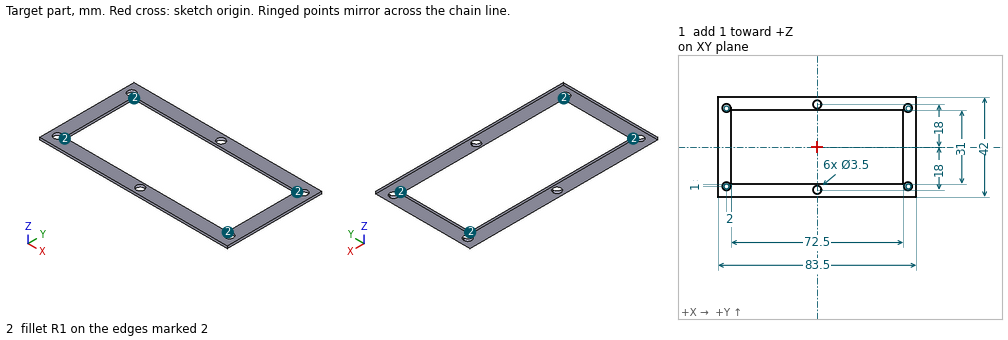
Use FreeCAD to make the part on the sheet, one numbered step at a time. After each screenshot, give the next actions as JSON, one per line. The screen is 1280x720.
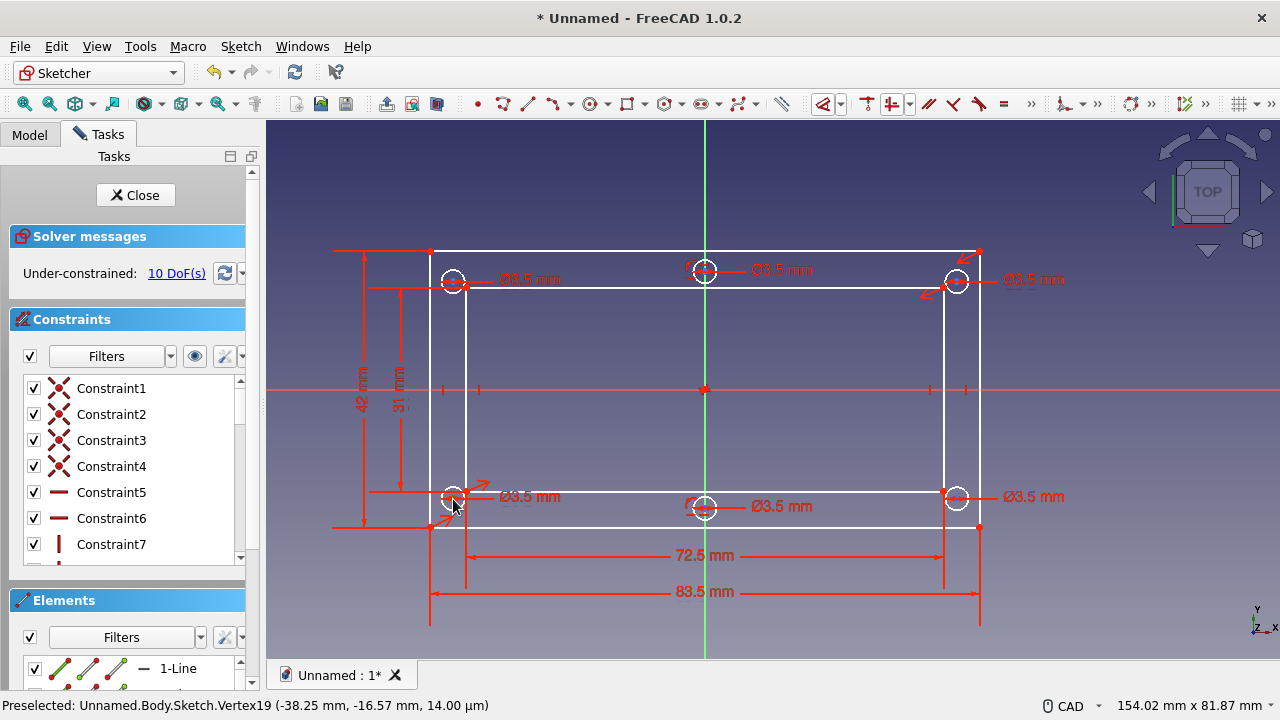
{"action": "left_click", "coordinate": [957, 499]}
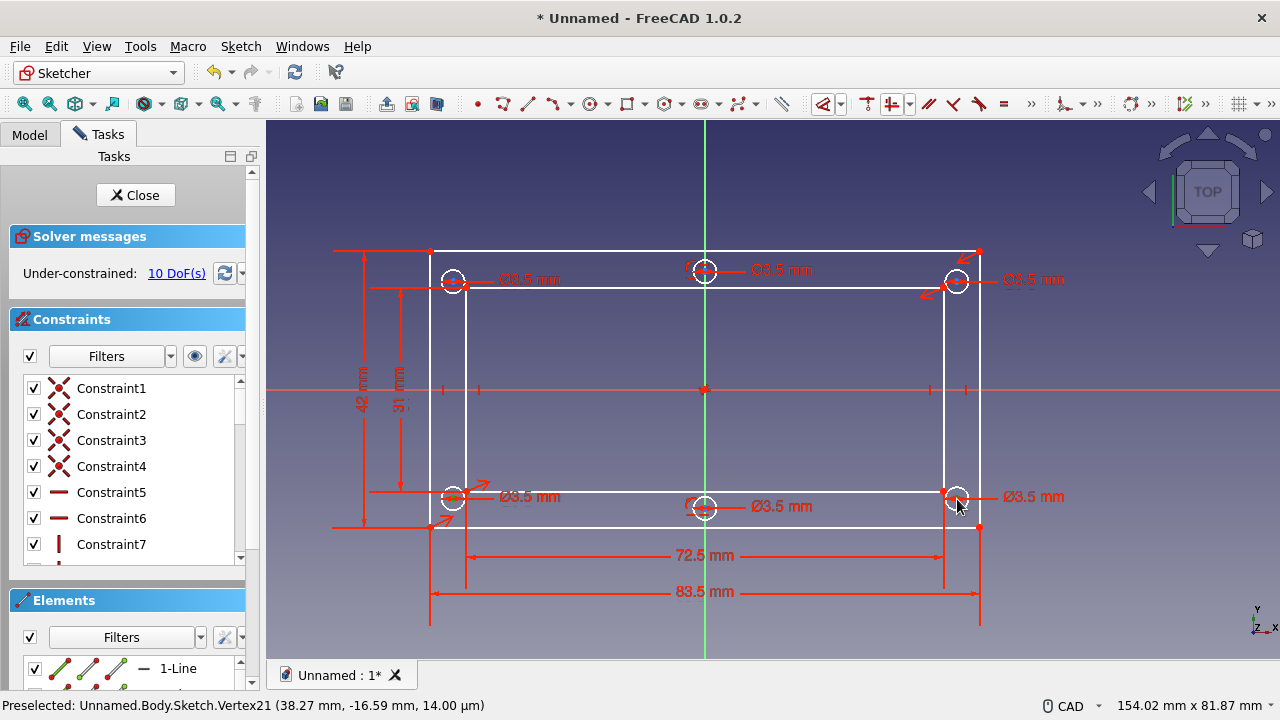
{"action": "left_click", "coordinate": [705, 458]}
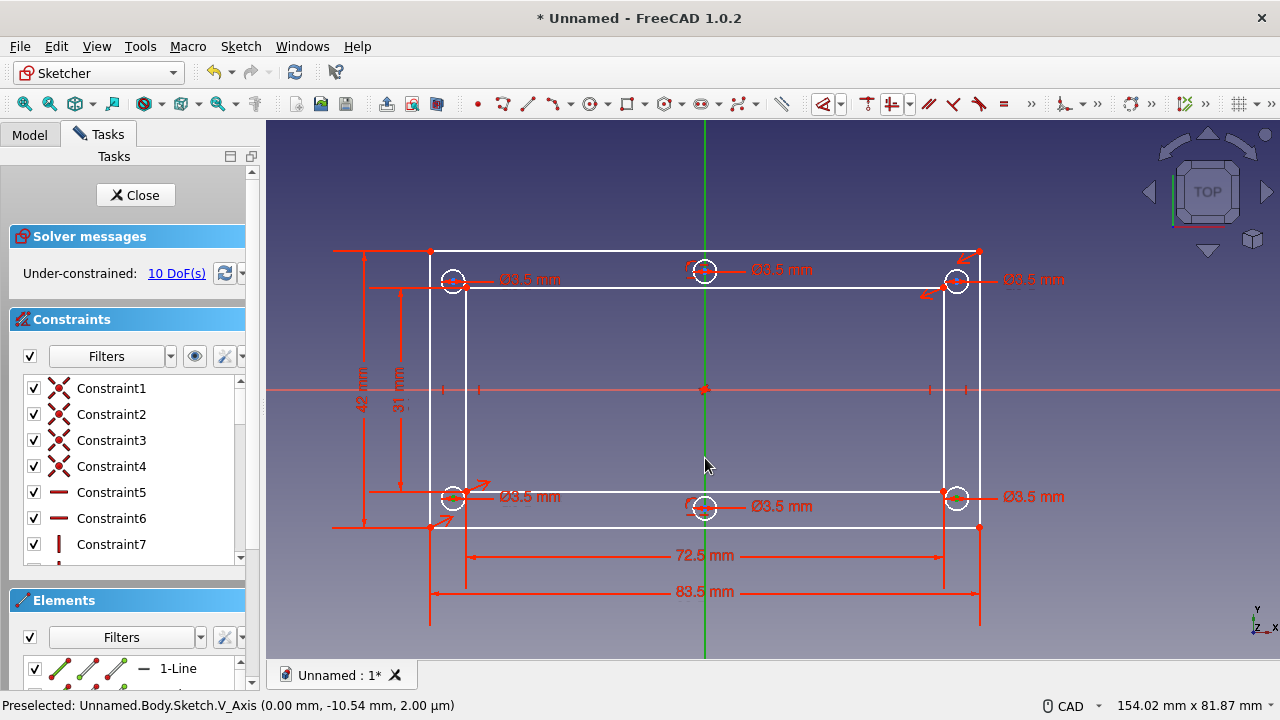
{"action": "key", "text": "s"}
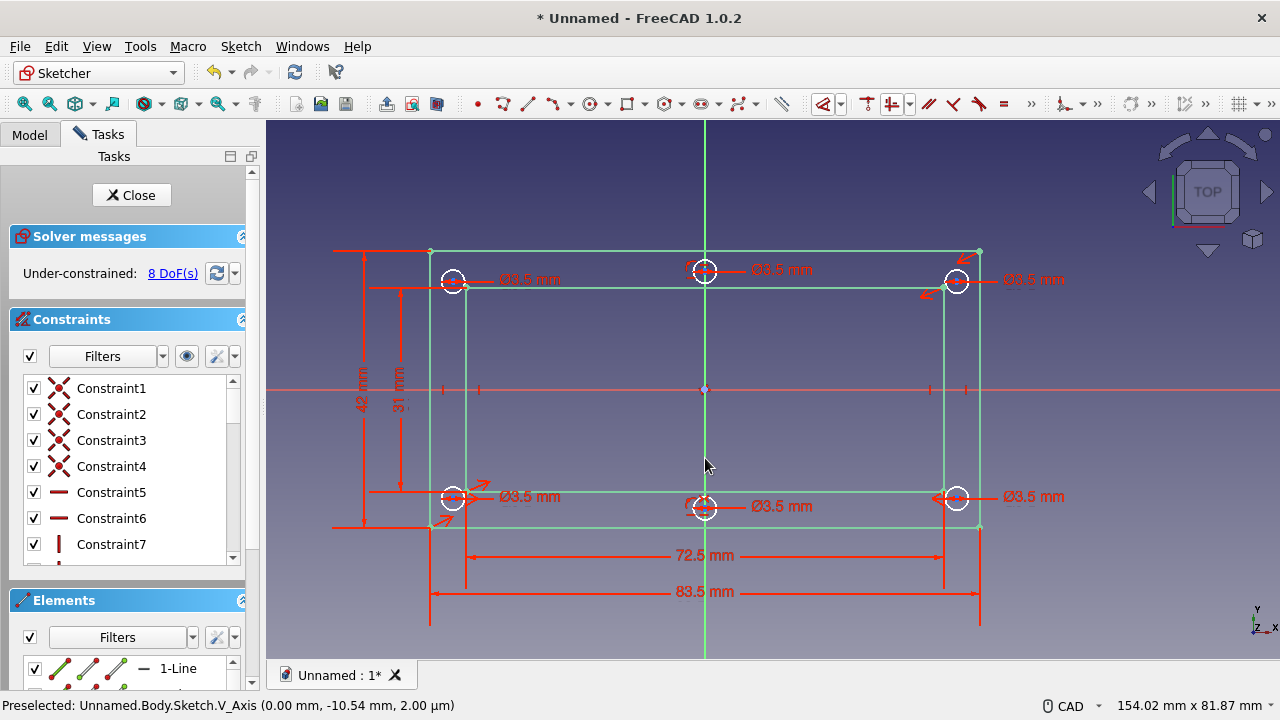
{"action": "left_click", "coordinate": [453, 499]}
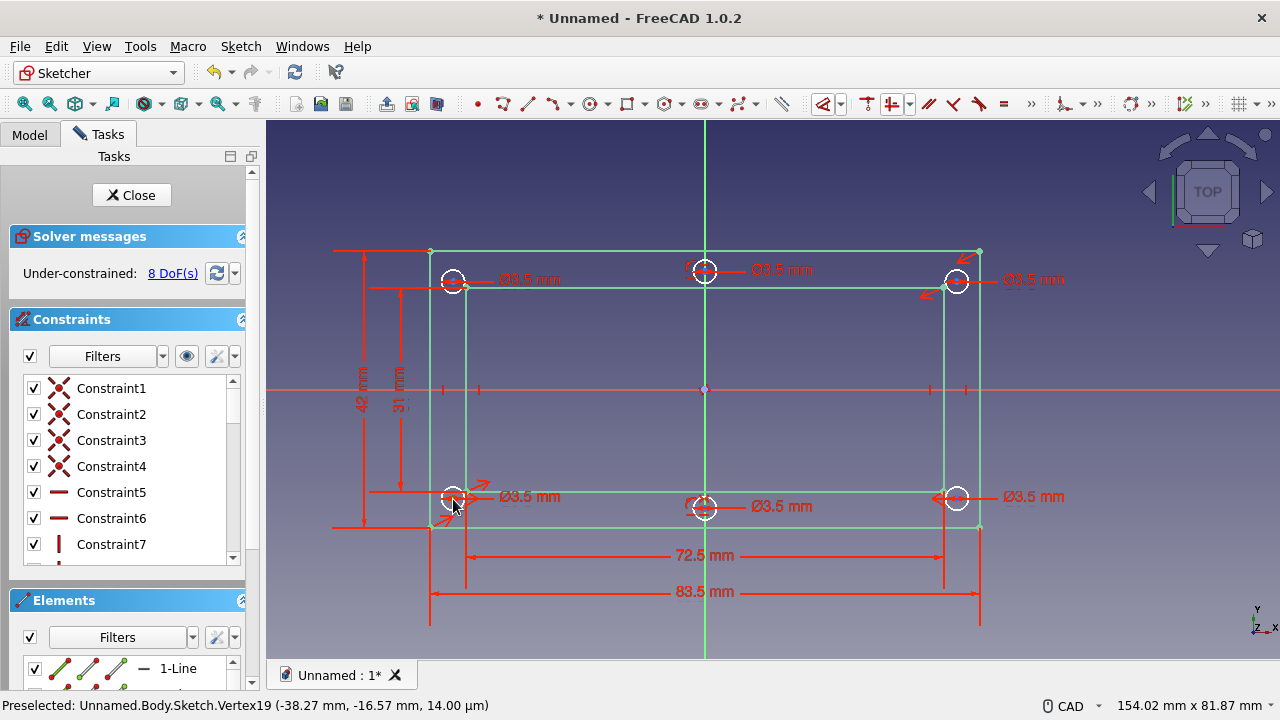
{"action": "left_click", "coordinate": [453, 282]}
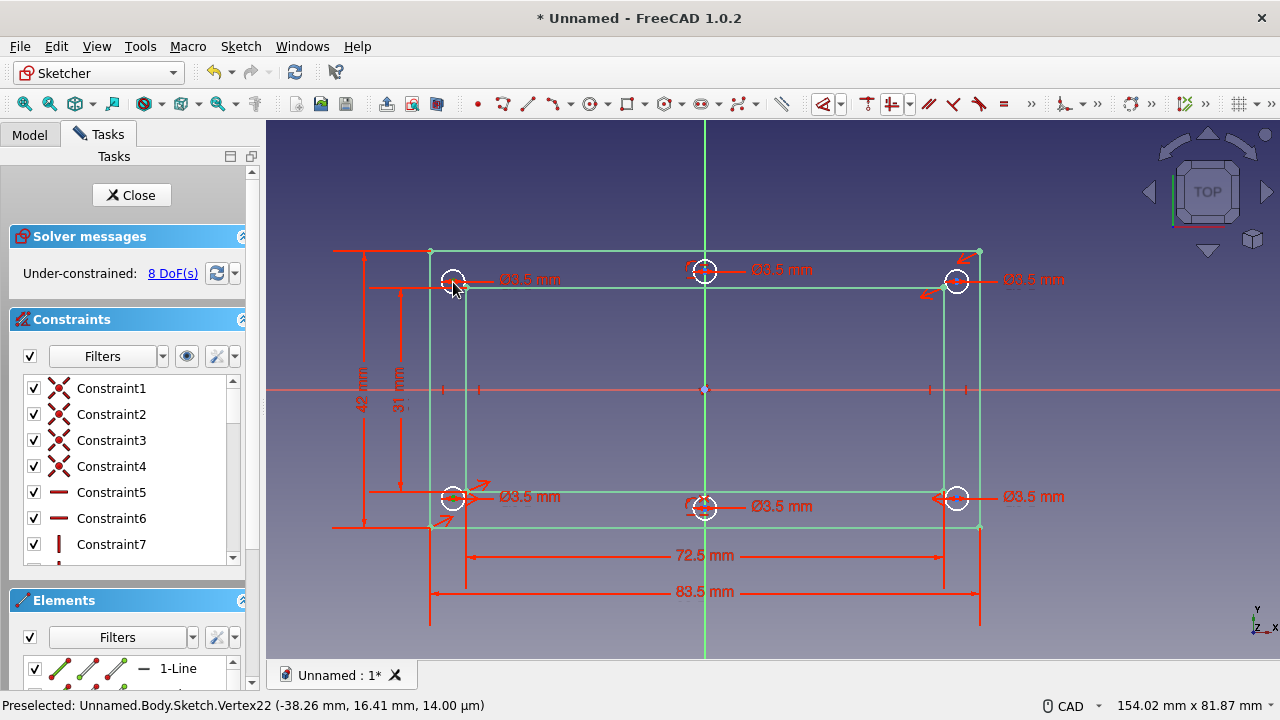
{"action": "left_click", "coordinate": [353, 390]}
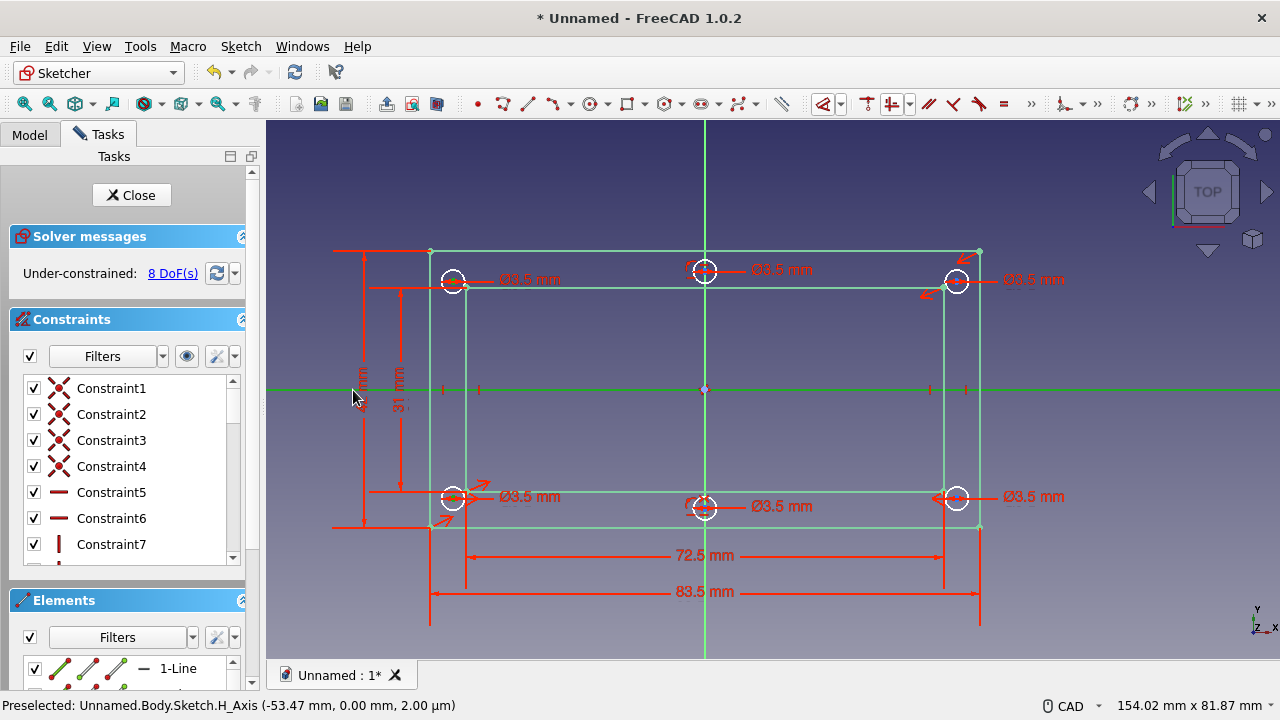
{"action": "key", "text": "s"}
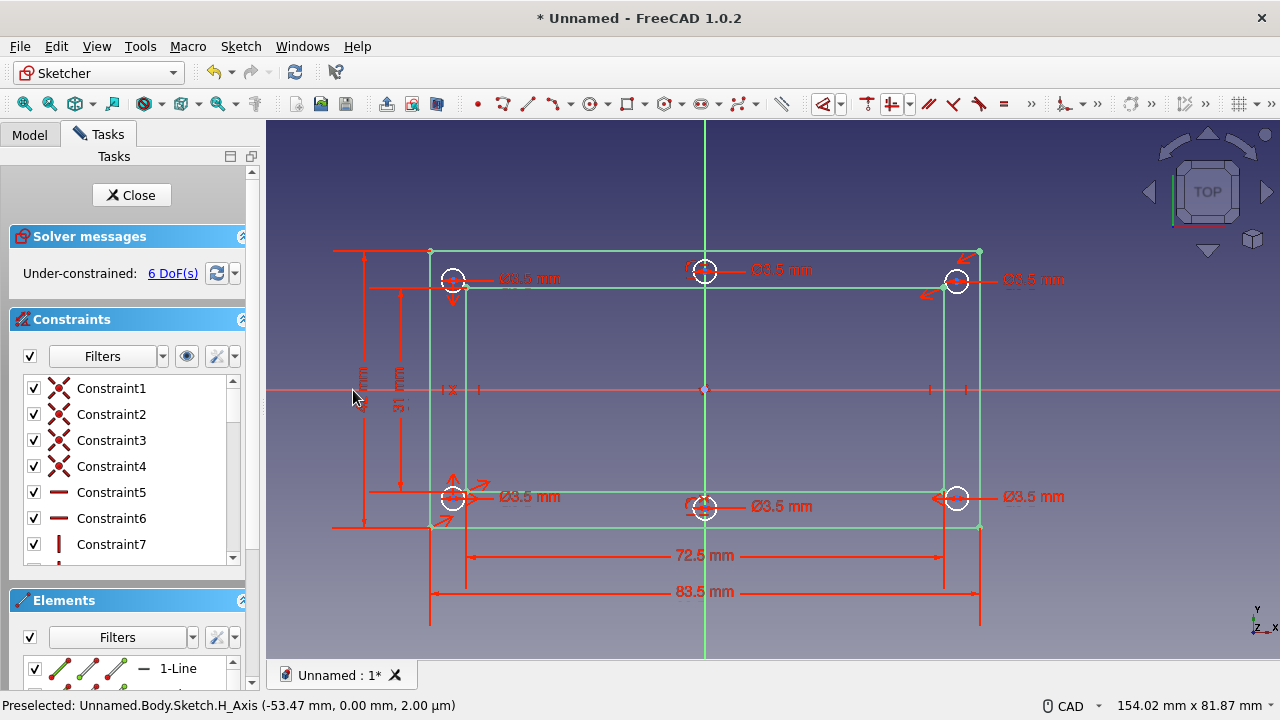
{"action": "left_click", "coordinate": [957, 499]}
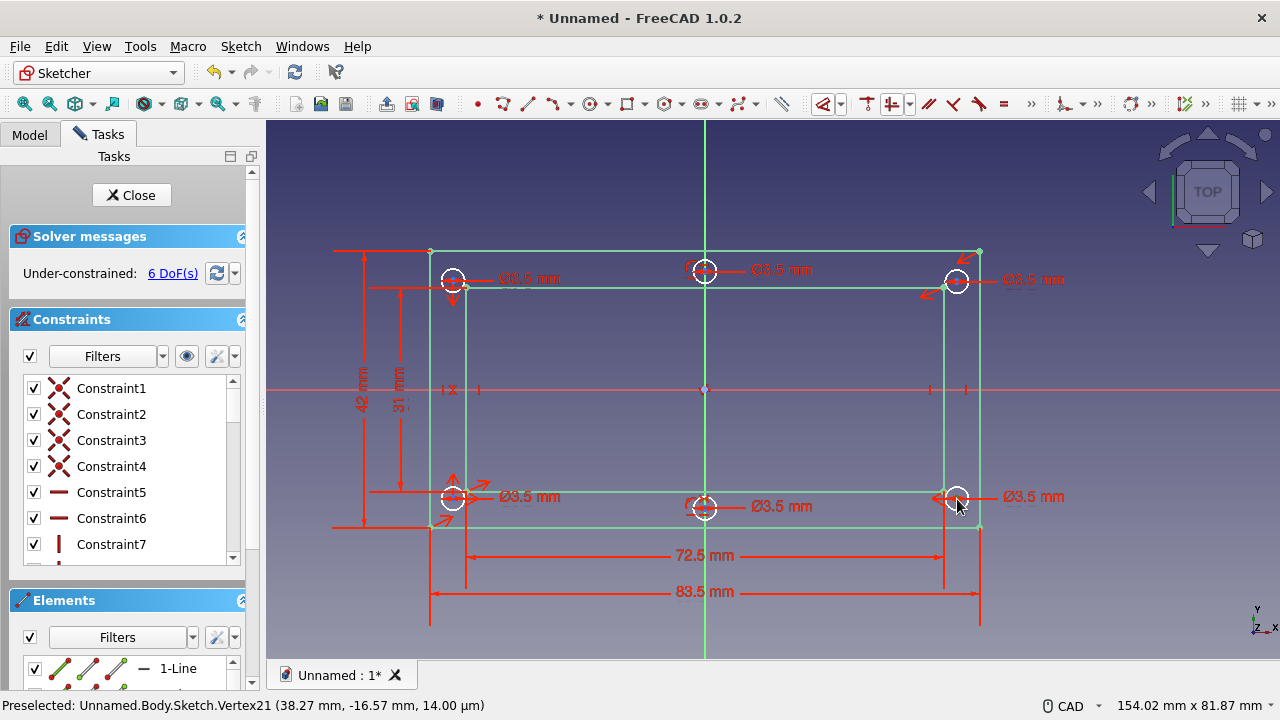
{"action": "left_click", "coordinate": [957, 282]}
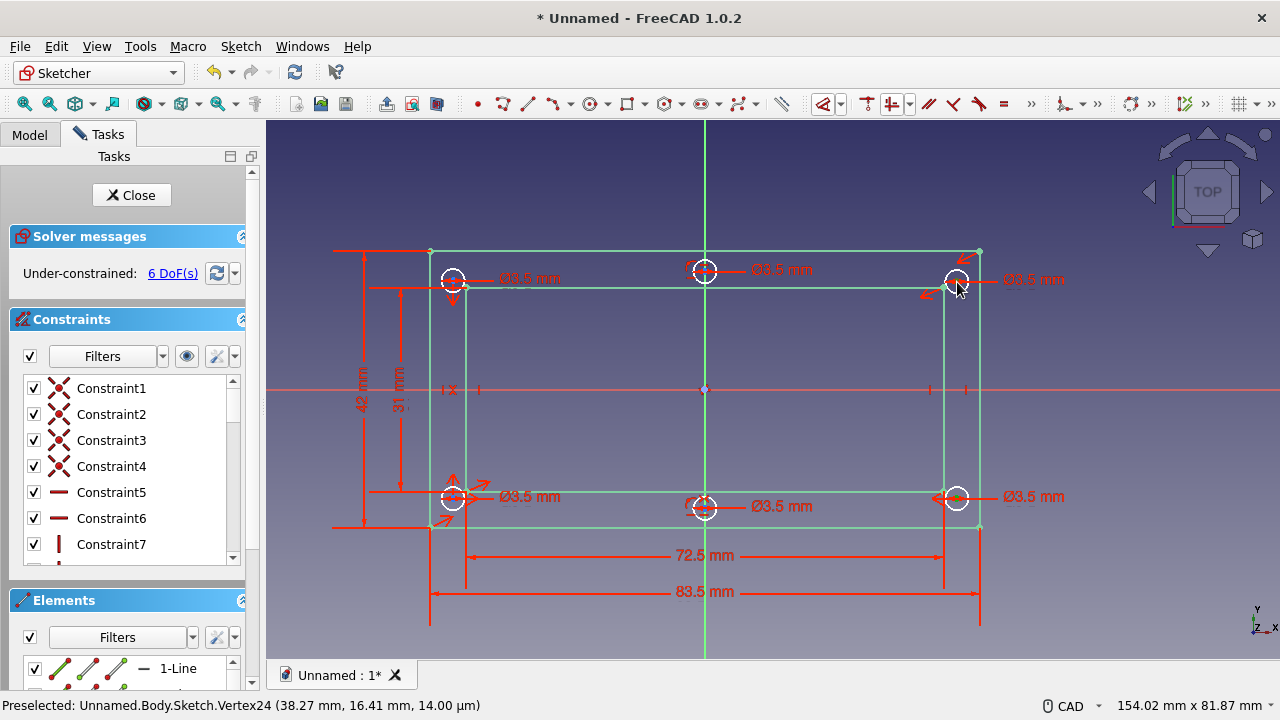
{"action": "left_click", "coordinate": [353, 390]}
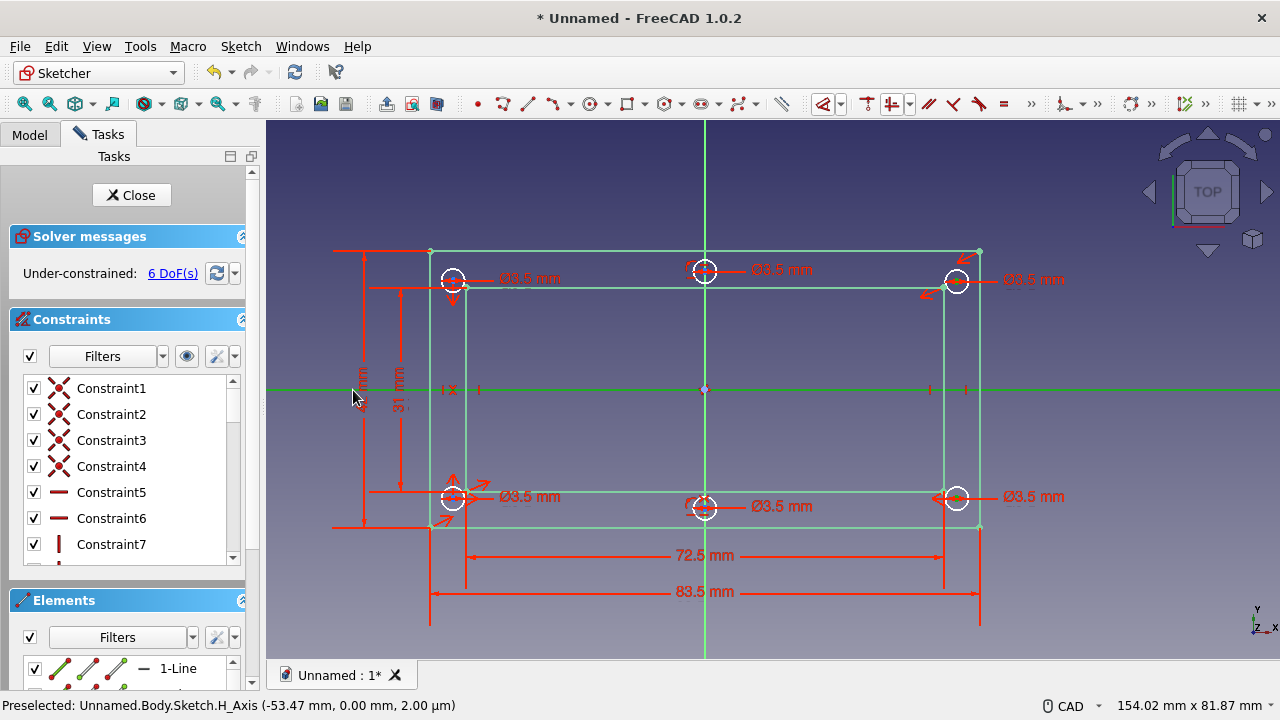
{"action": "key", "text": "s"}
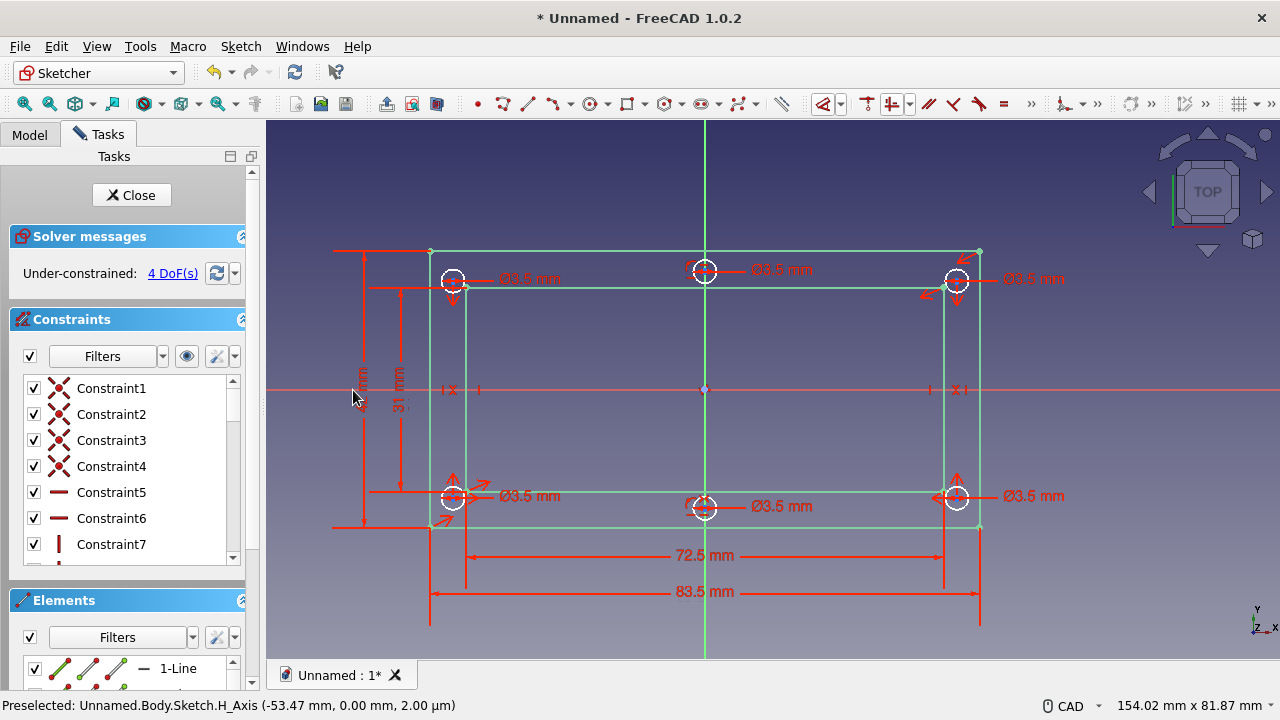
{"action": "left_click", "coordinate": [822, 104]}